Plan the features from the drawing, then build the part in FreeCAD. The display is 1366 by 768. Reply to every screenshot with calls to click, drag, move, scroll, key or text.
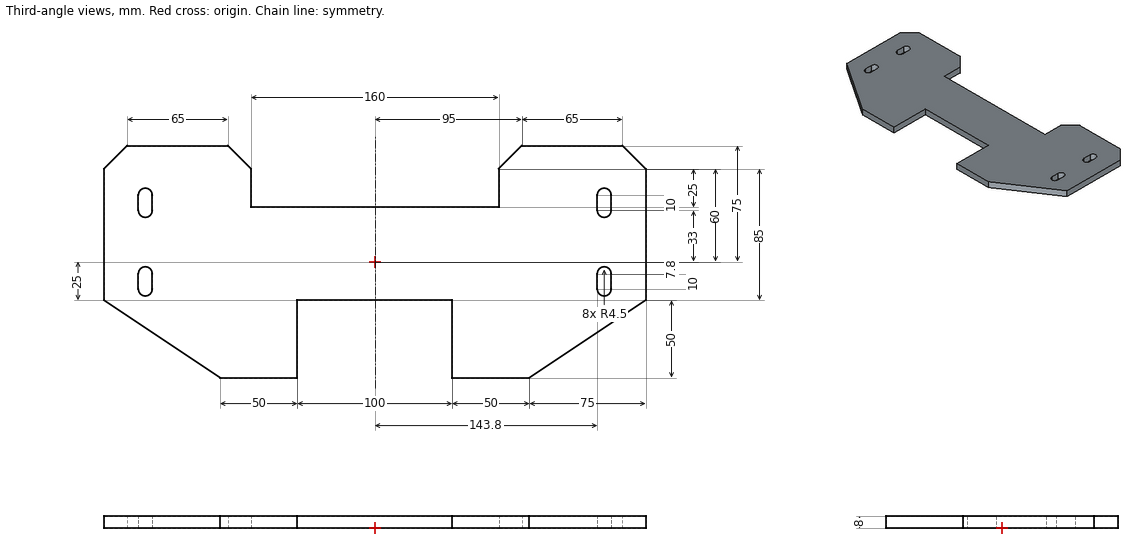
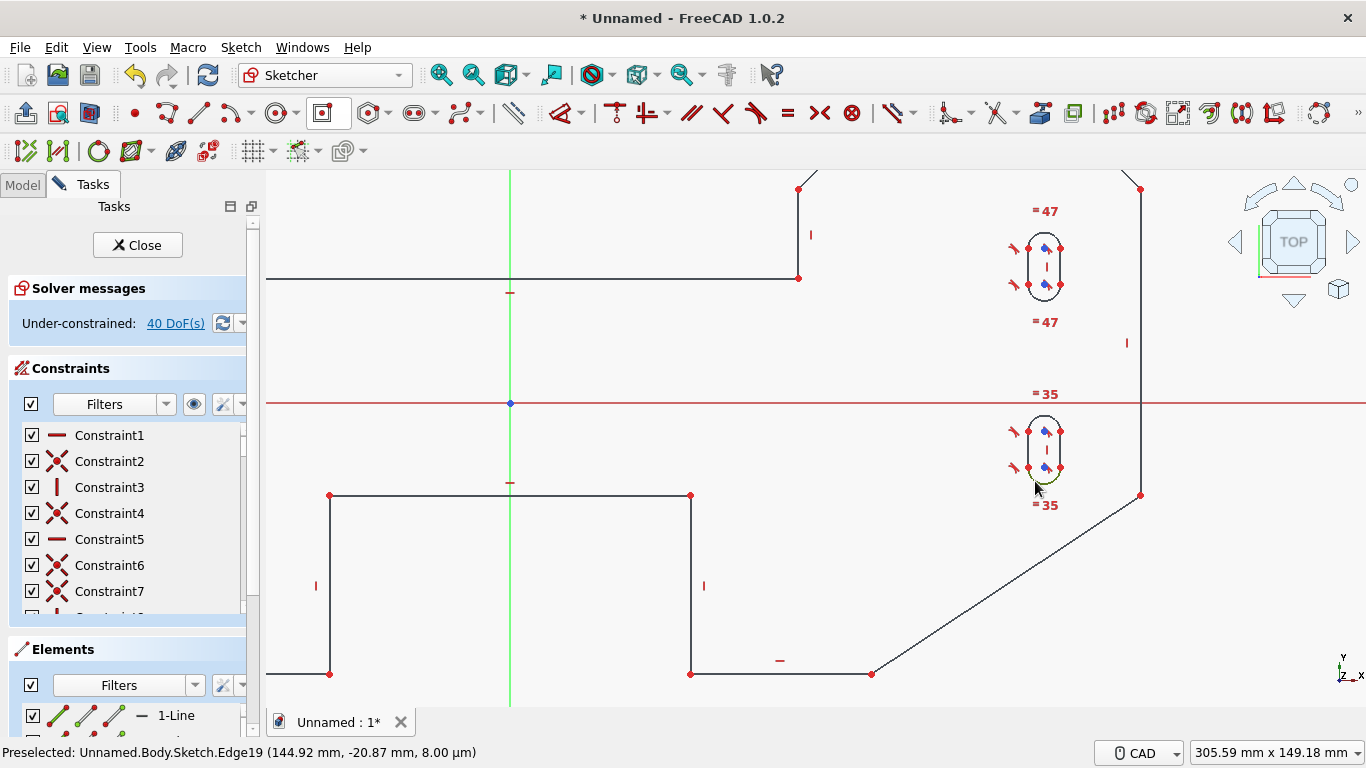
scroll(1036, 482, down, 3)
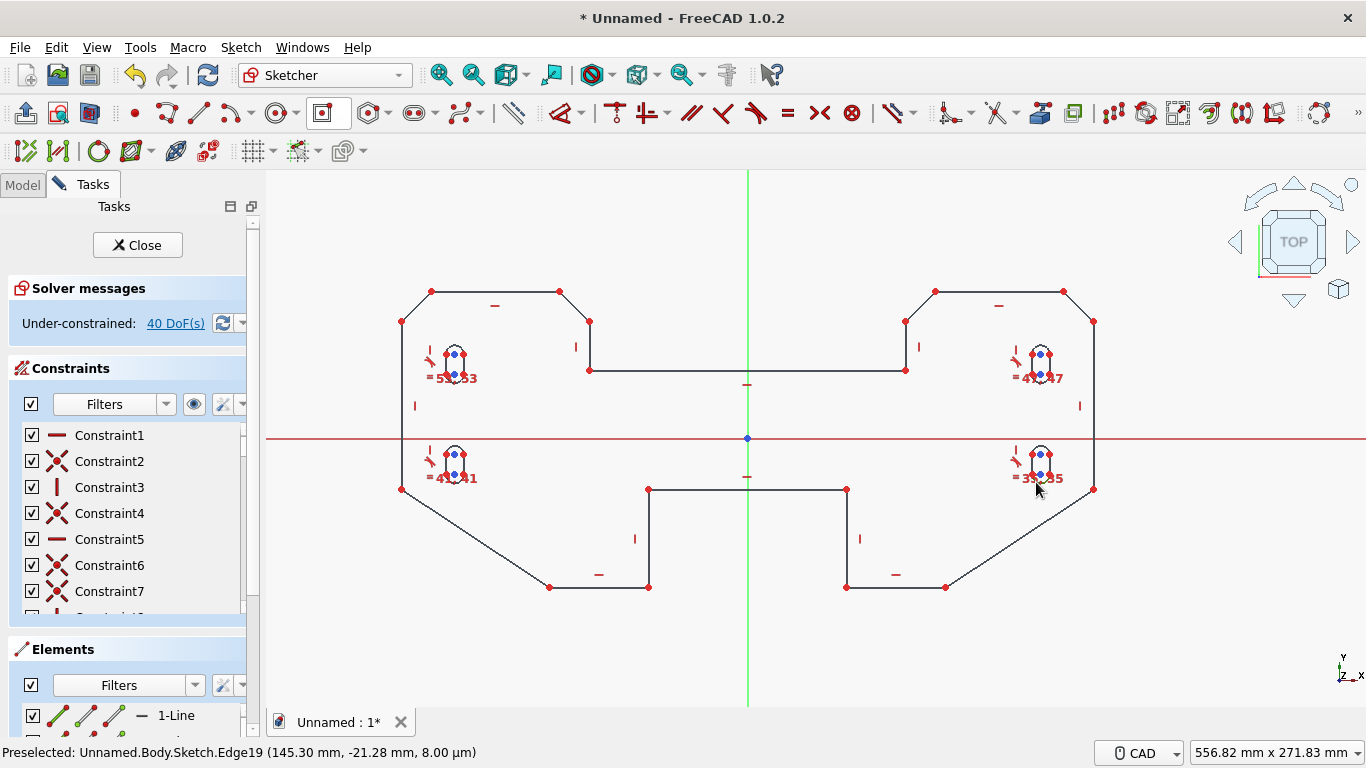
scroll(450, 482, up, 3)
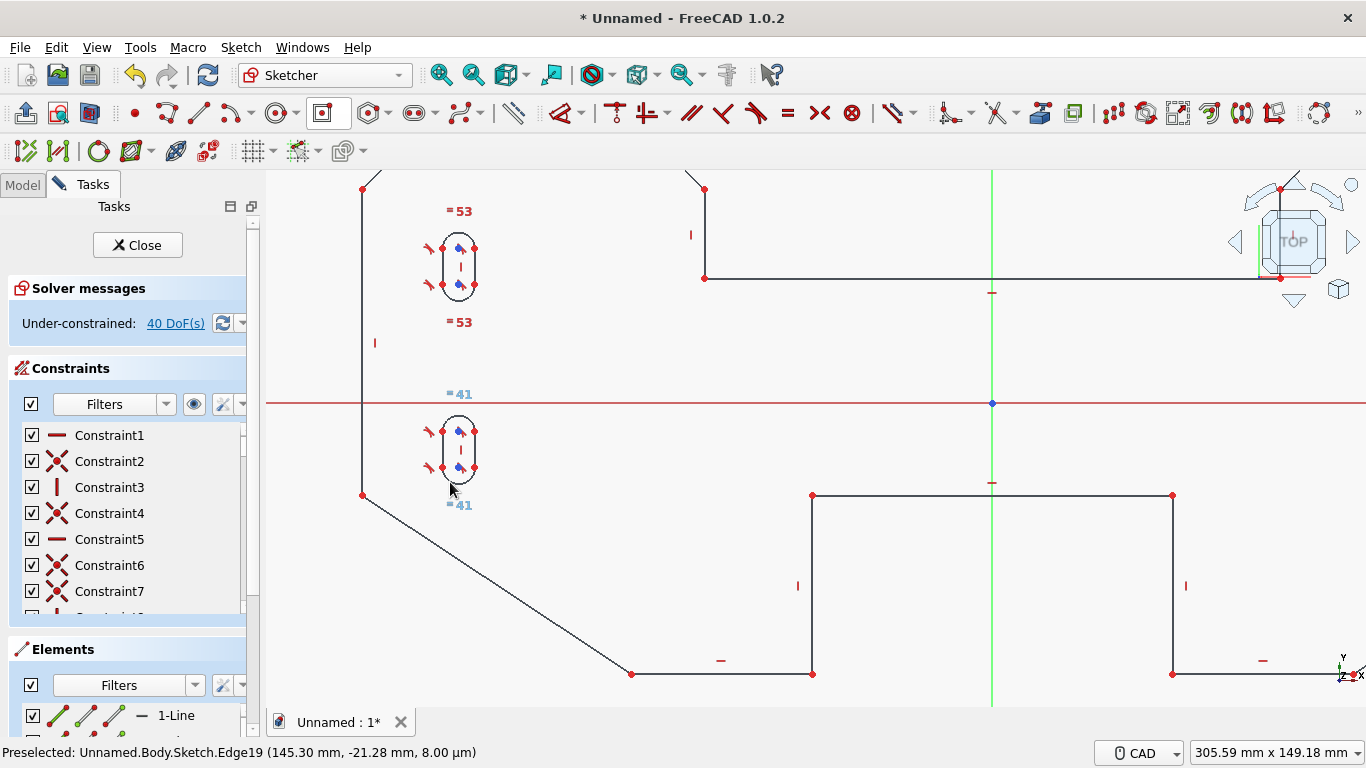
click(449, 481)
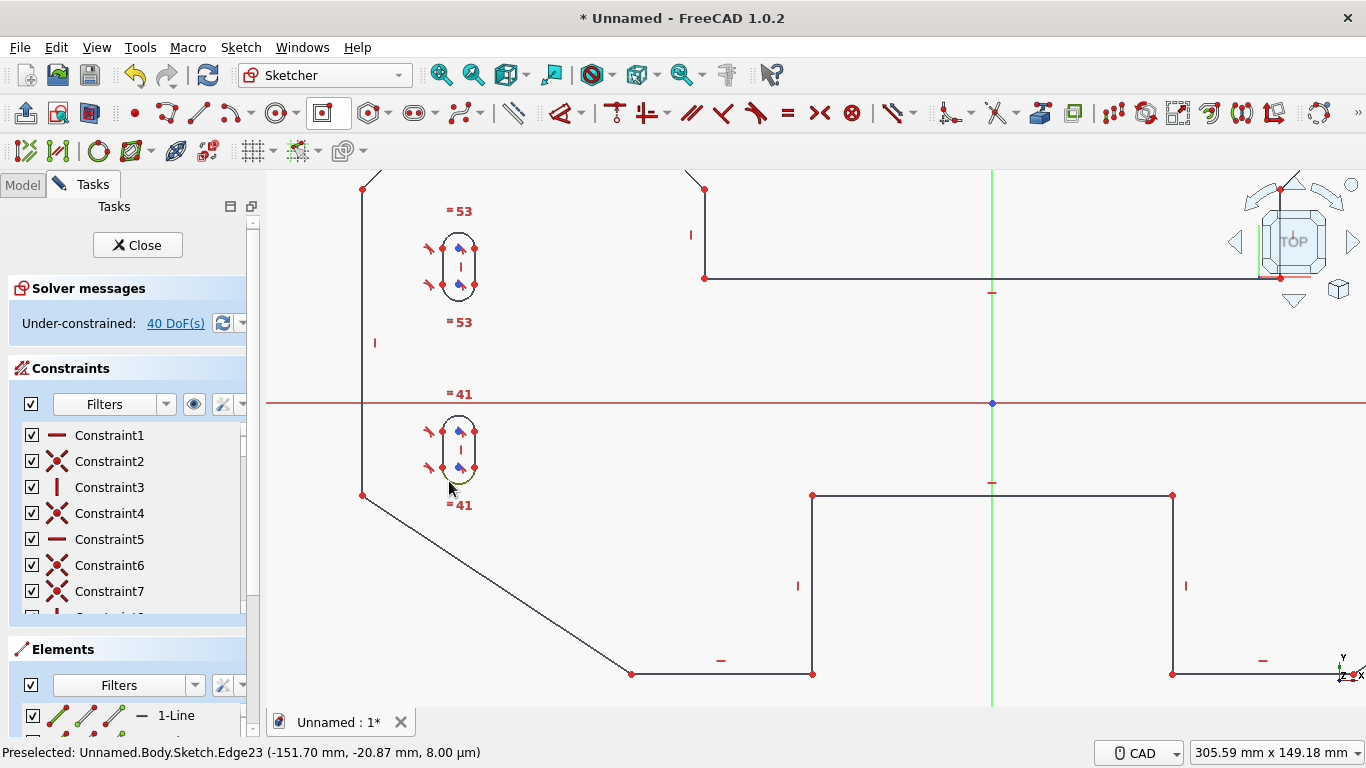
scroll(449, 482, down, 3)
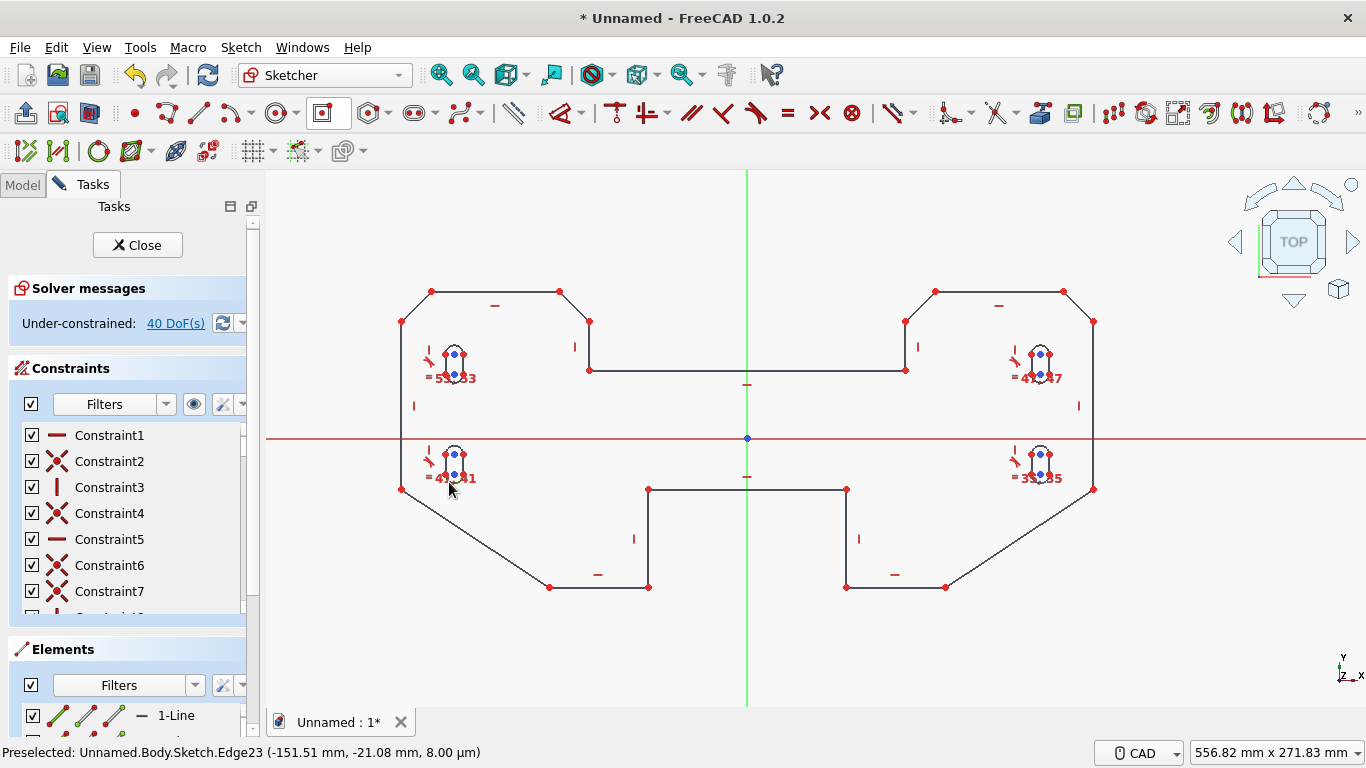
scroll(1035, 381, up, 3)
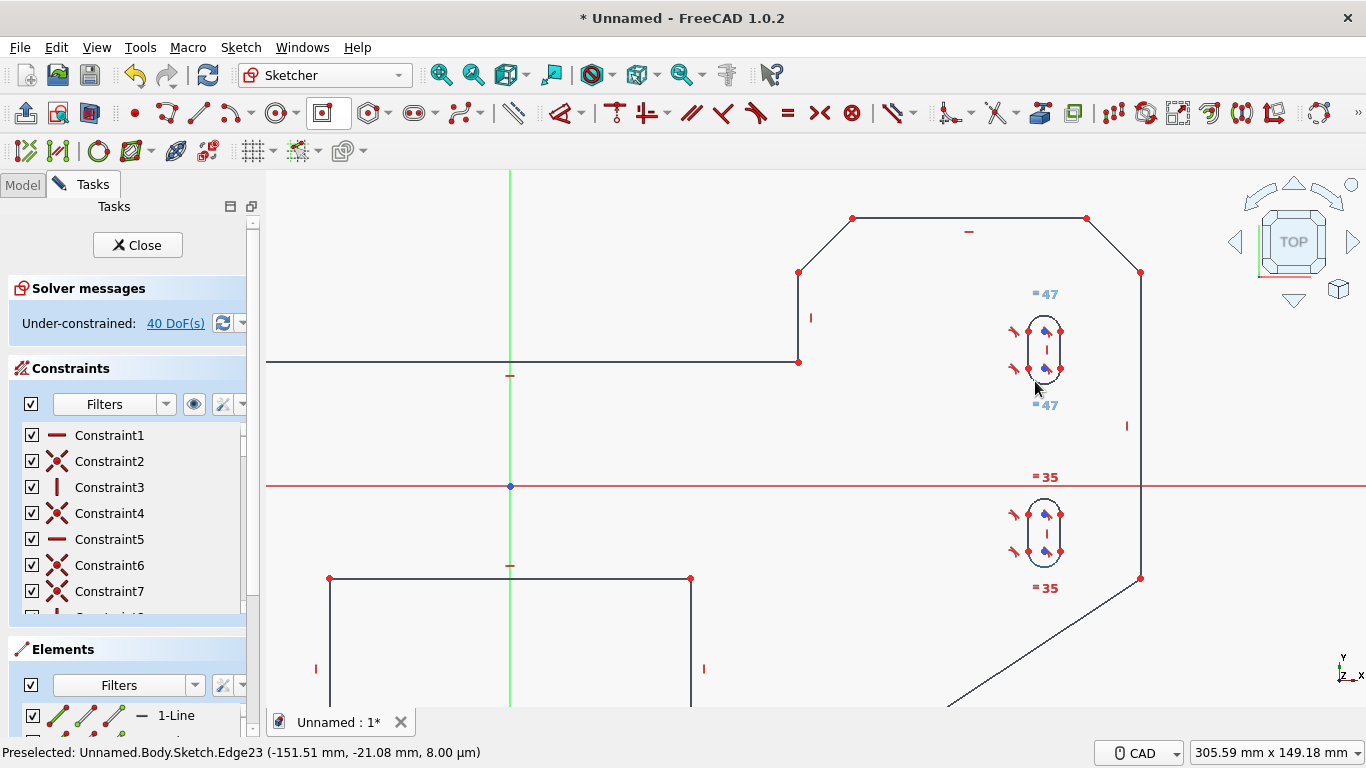
click(1035, 381)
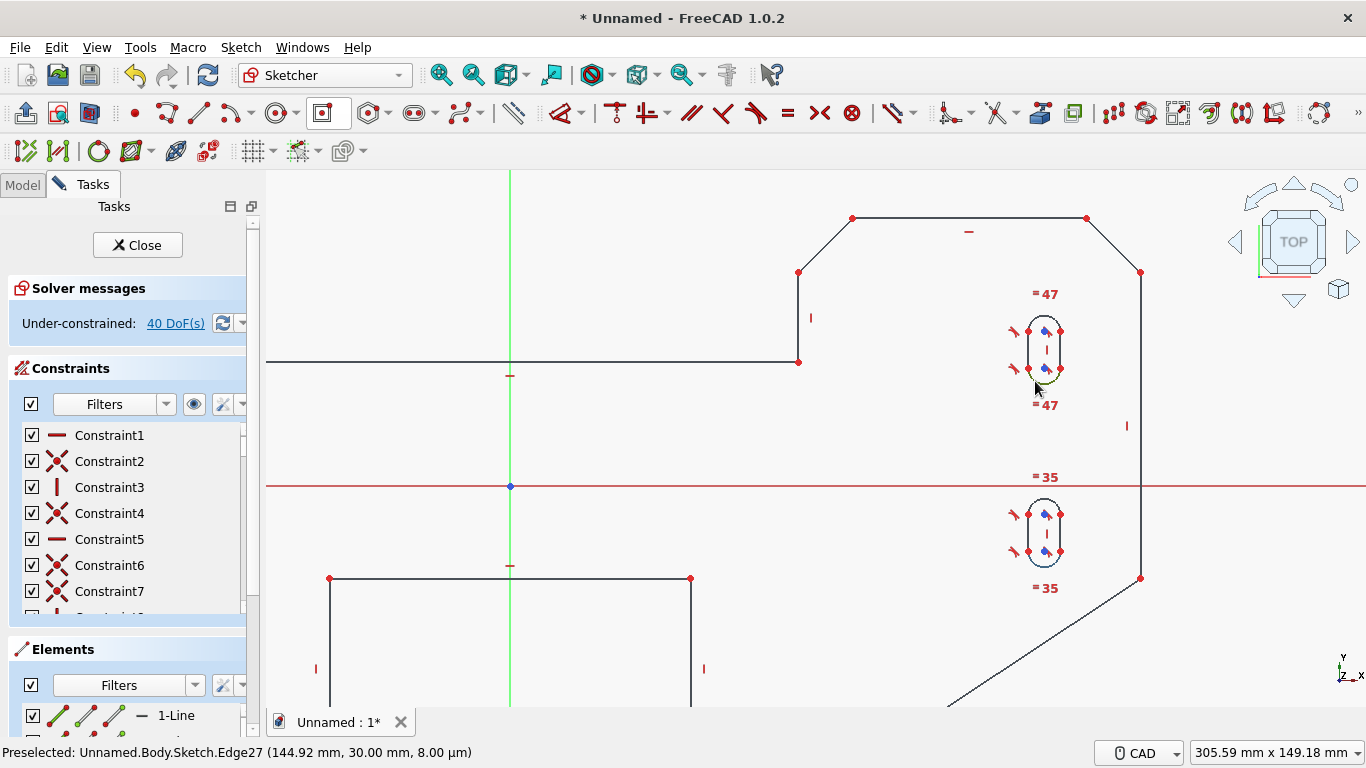
scroll(1036, 380, down, 3)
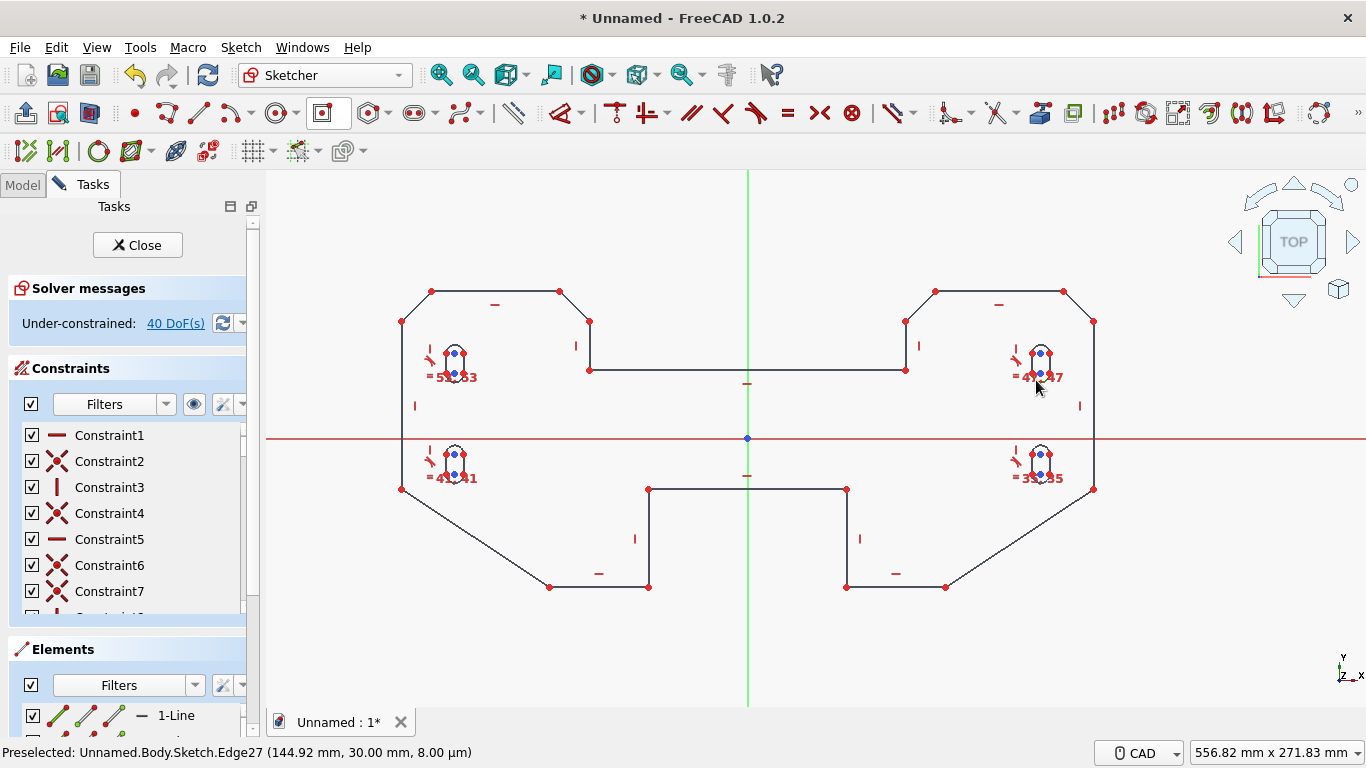
scroll(450, 381, up, 3)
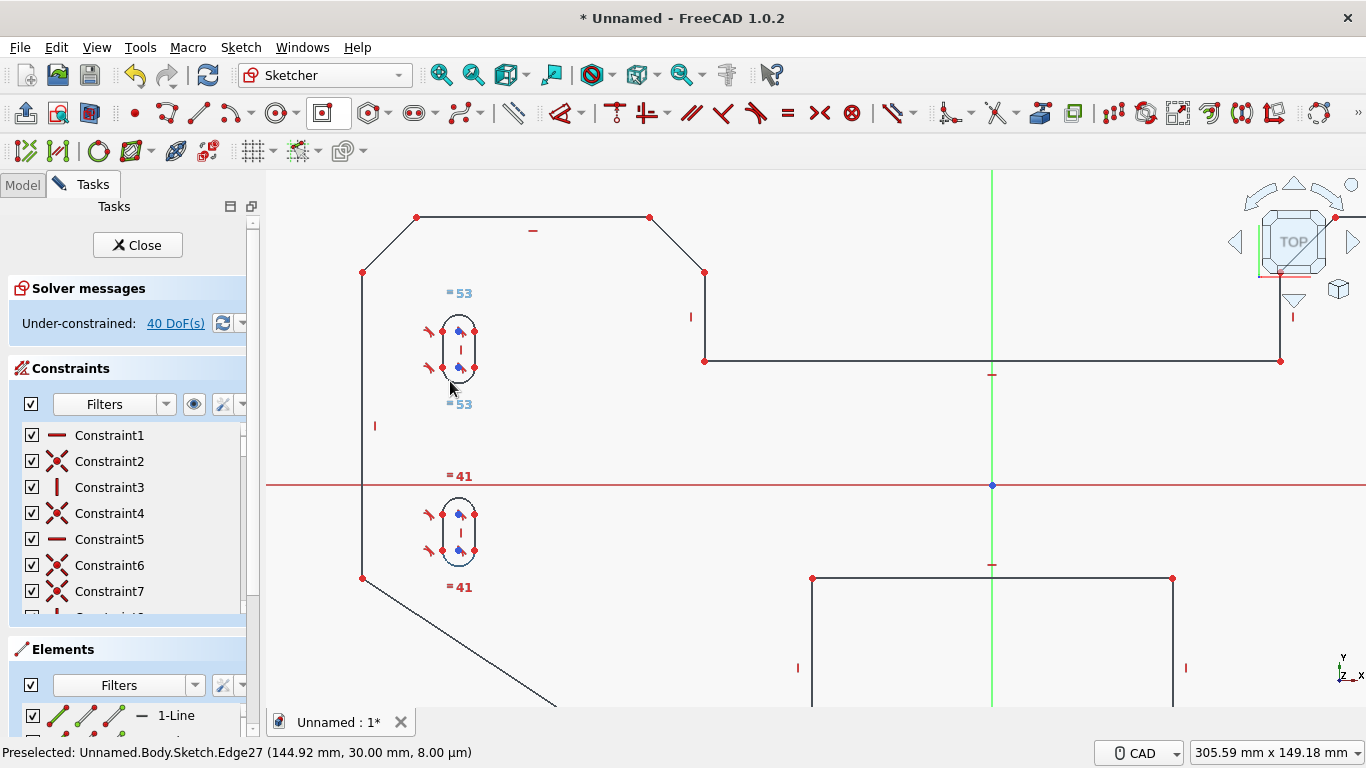
click(449, 380)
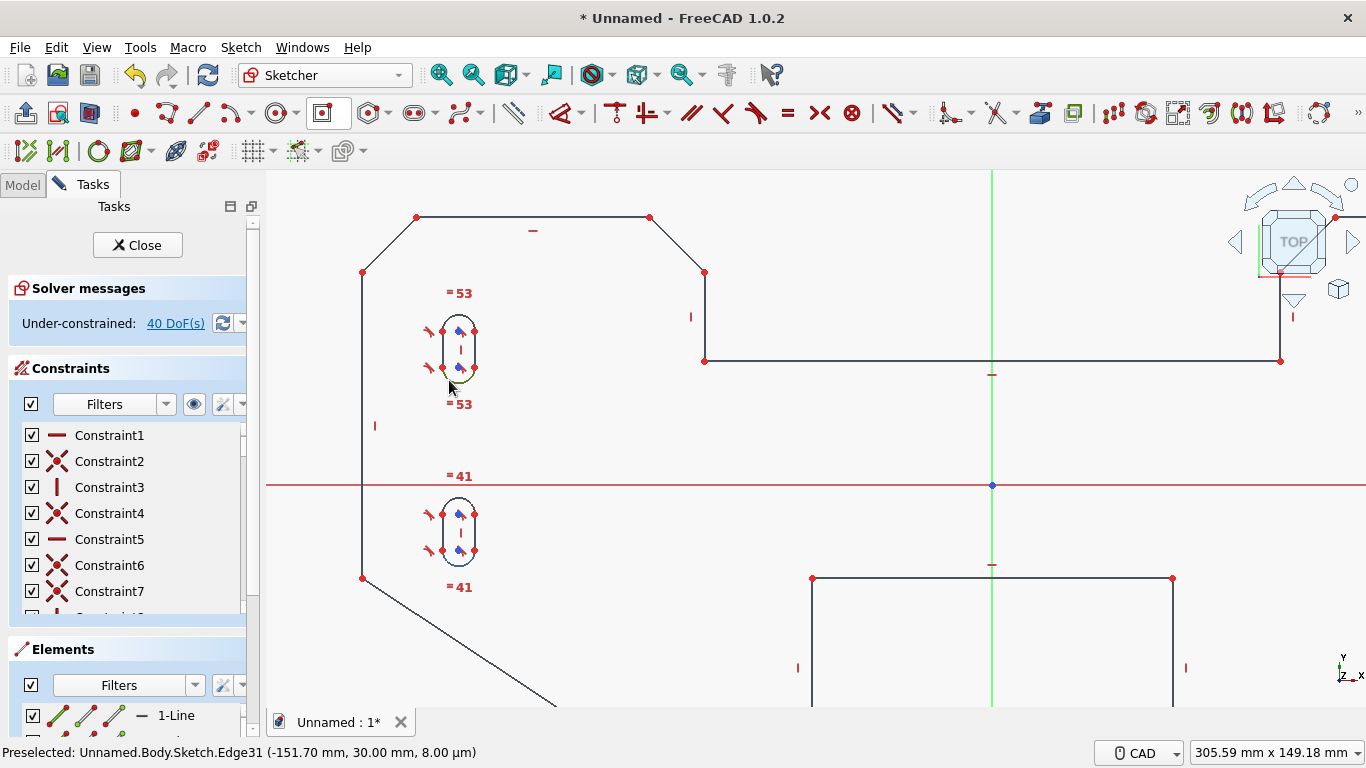
click(788, 114)